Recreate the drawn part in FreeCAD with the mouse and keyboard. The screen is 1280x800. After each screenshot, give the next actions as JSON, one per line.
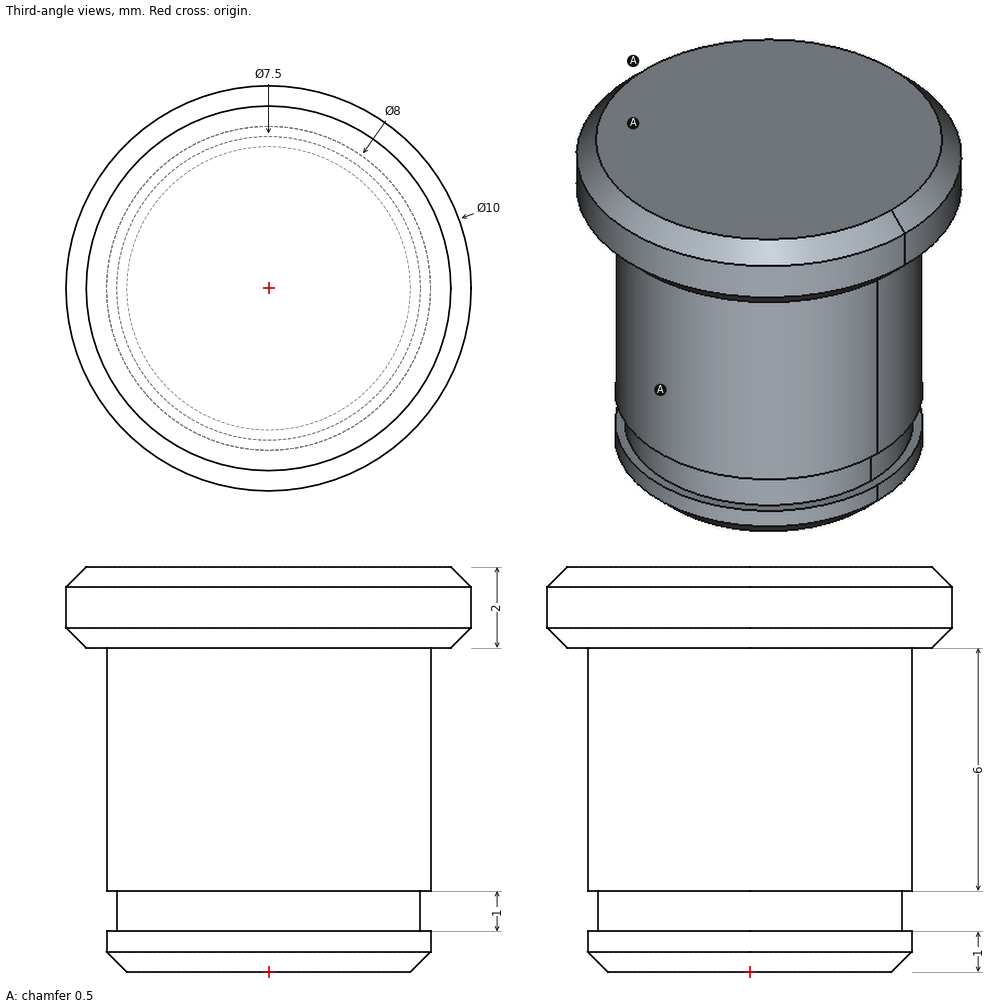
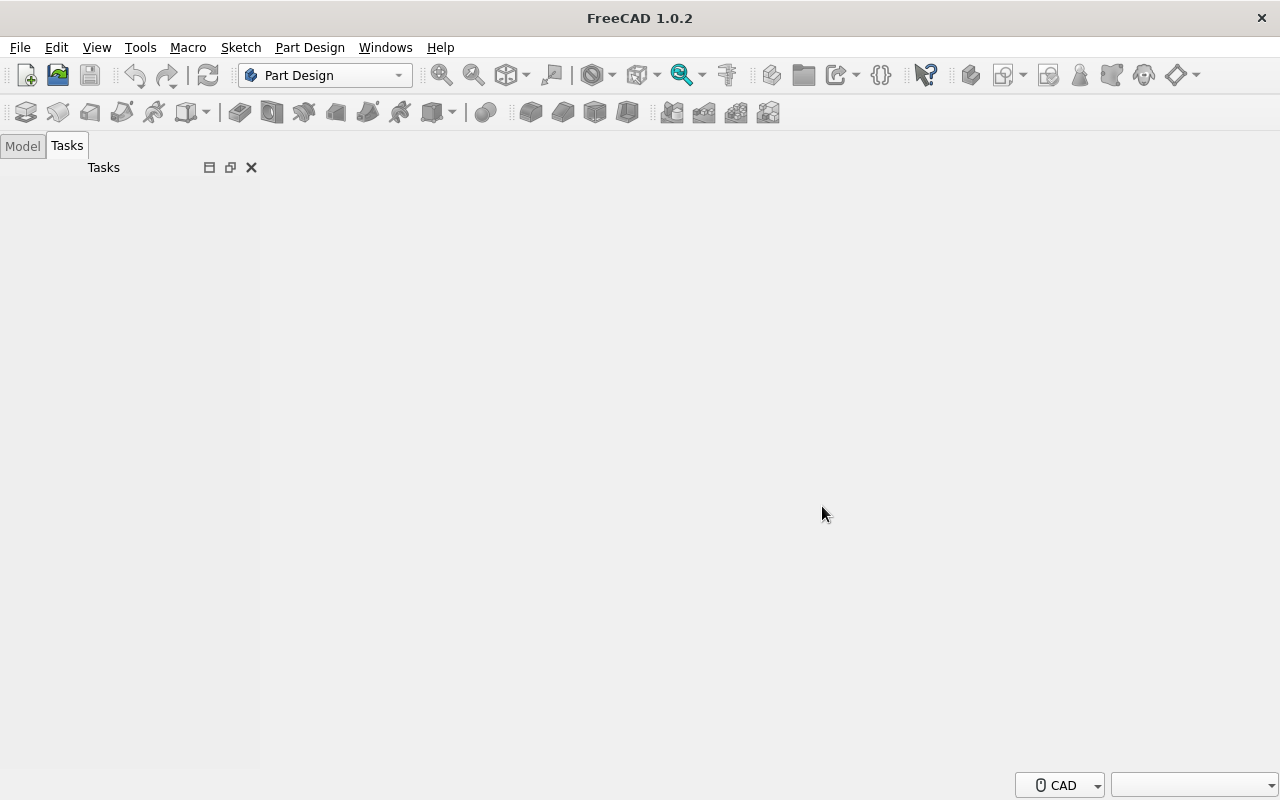
{"action": "key", "text": "ctrl+n"}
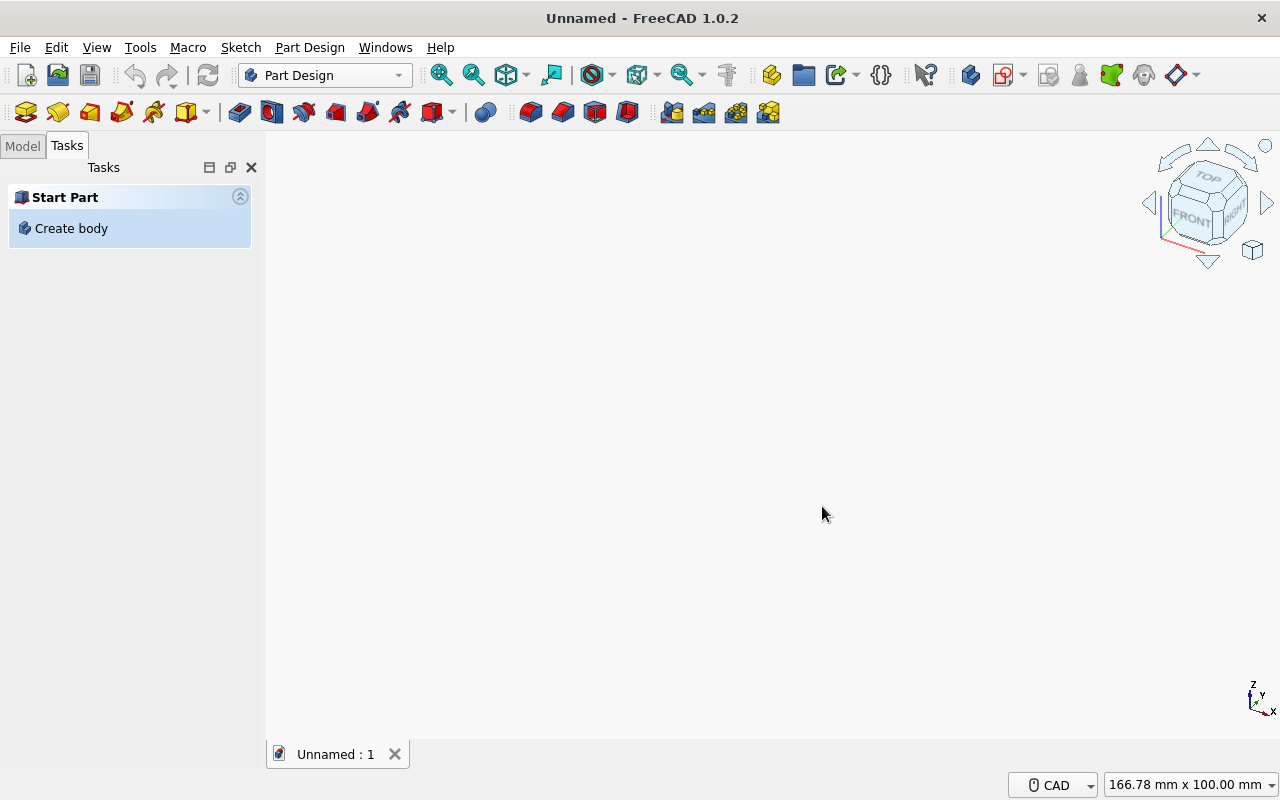
{"action": "left_click", "coordinate": [1004, 76]}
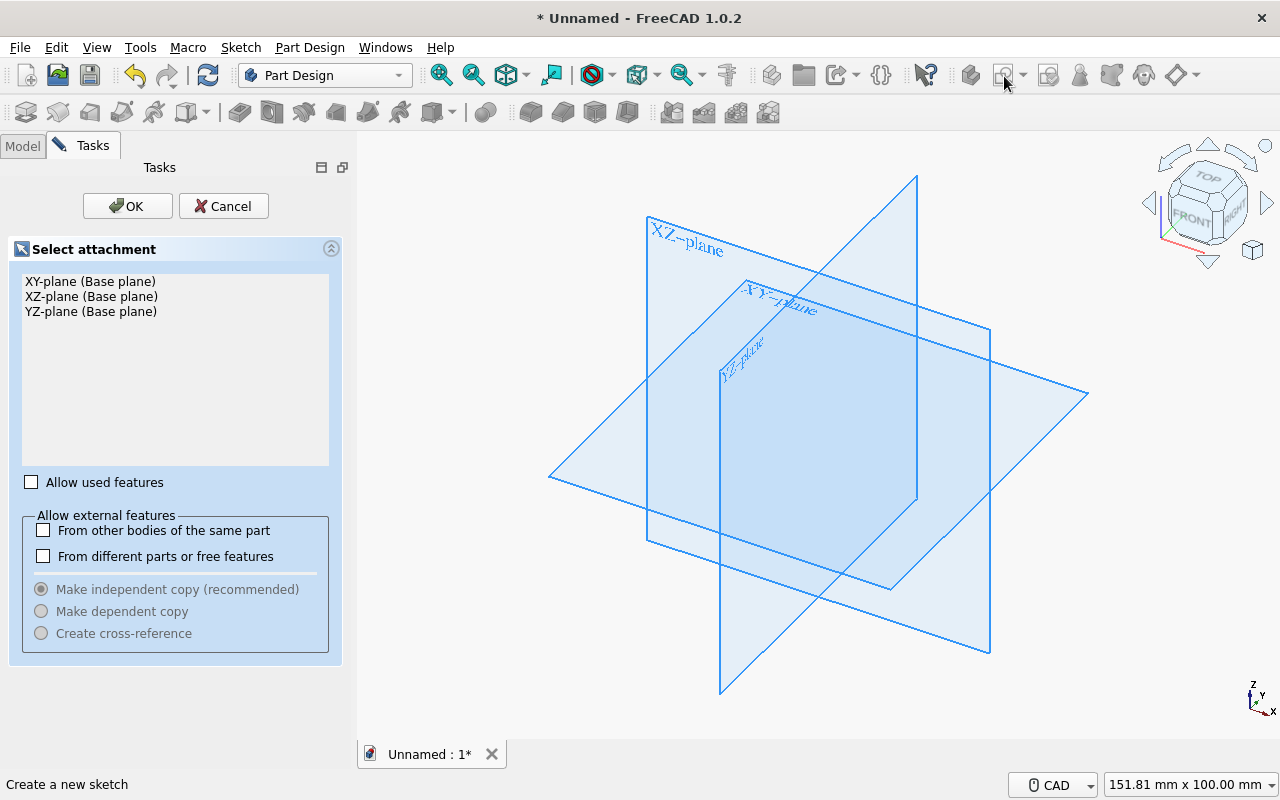
{"action": "left_click", "coordinate": [82, 282]}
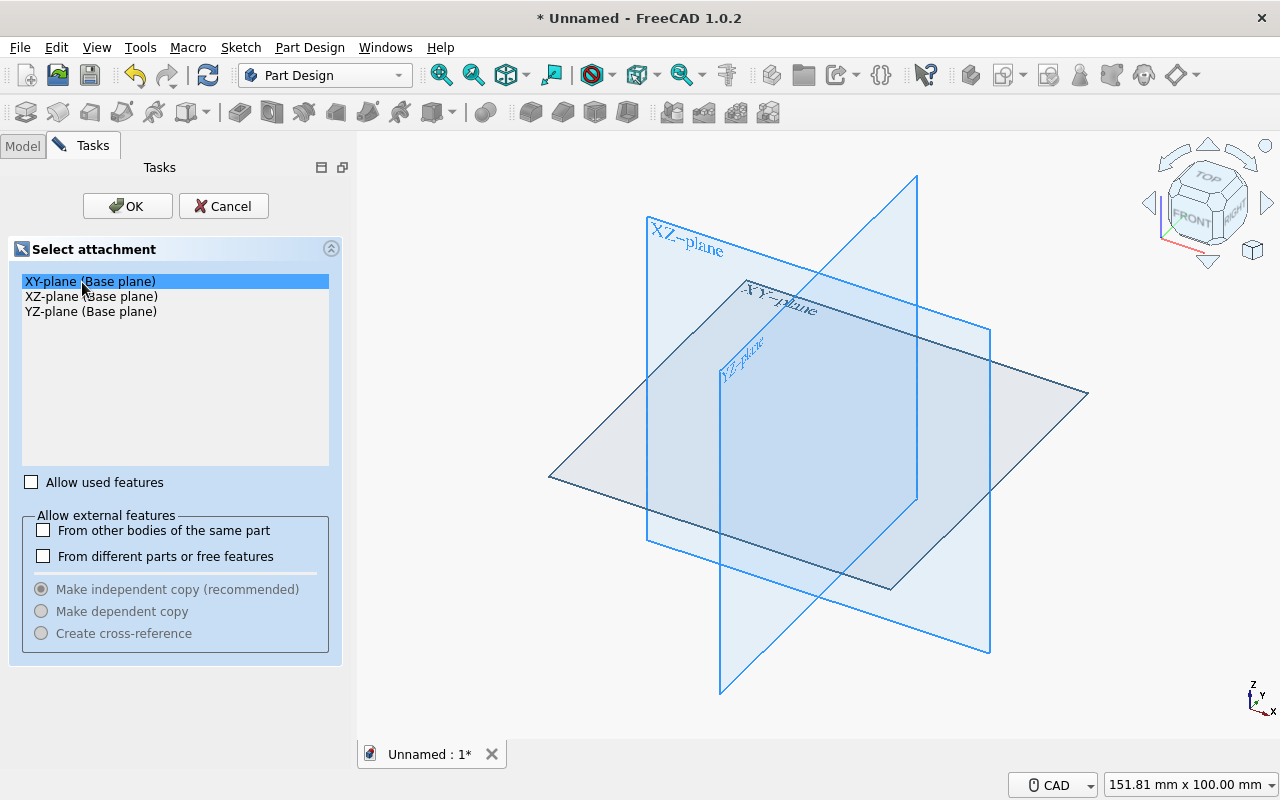
{"action": "left_click", "coordinate": [128, 206]}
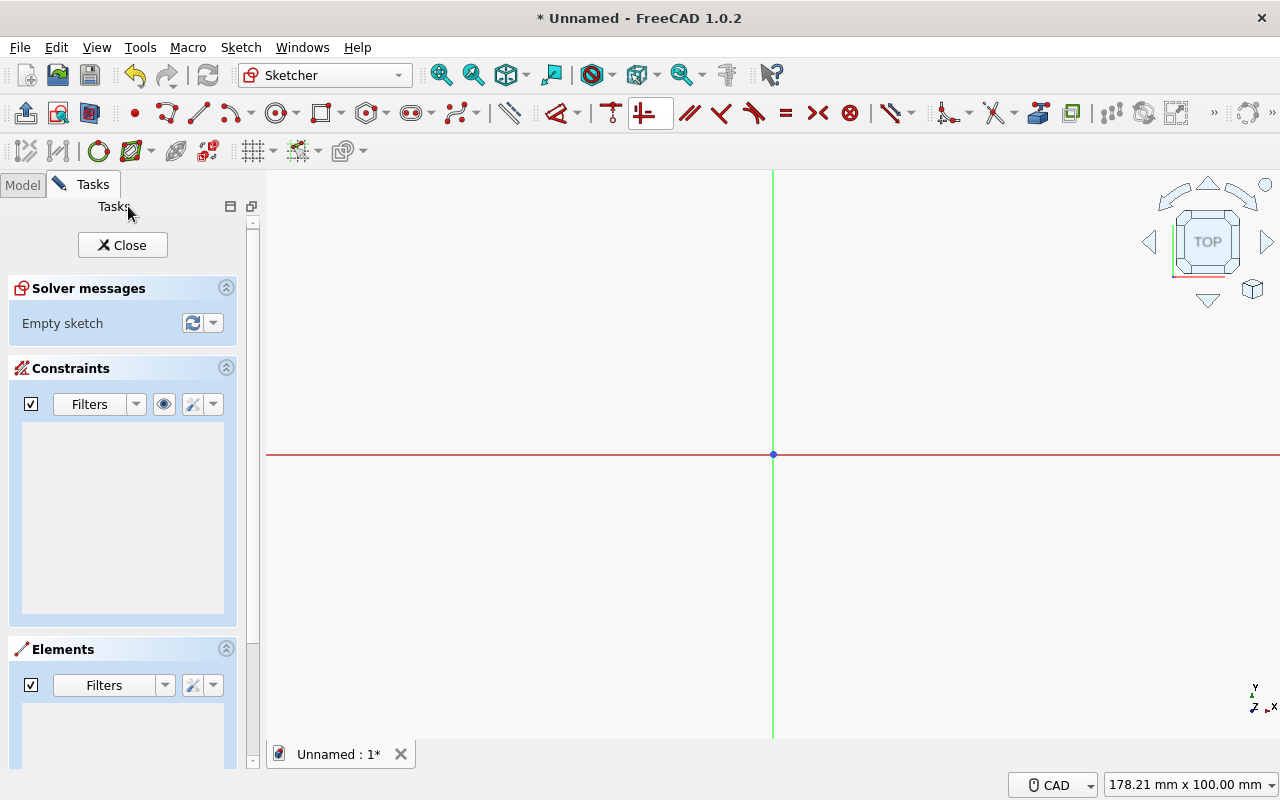
{"action": "scroll", "coordinate": [784, 454], "scroll_direction": "up", "scroll_amount": 10}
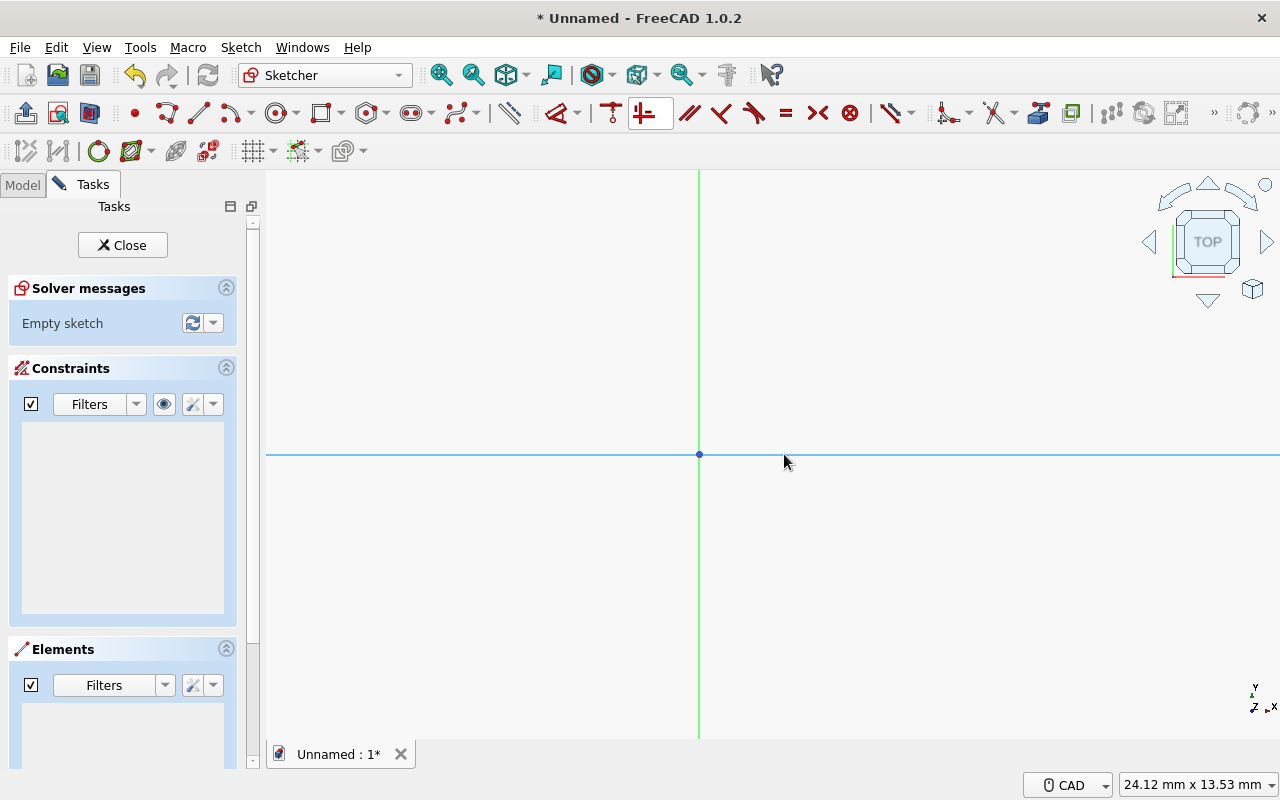
{"action": "left_click", "coordinate": [276, 114]}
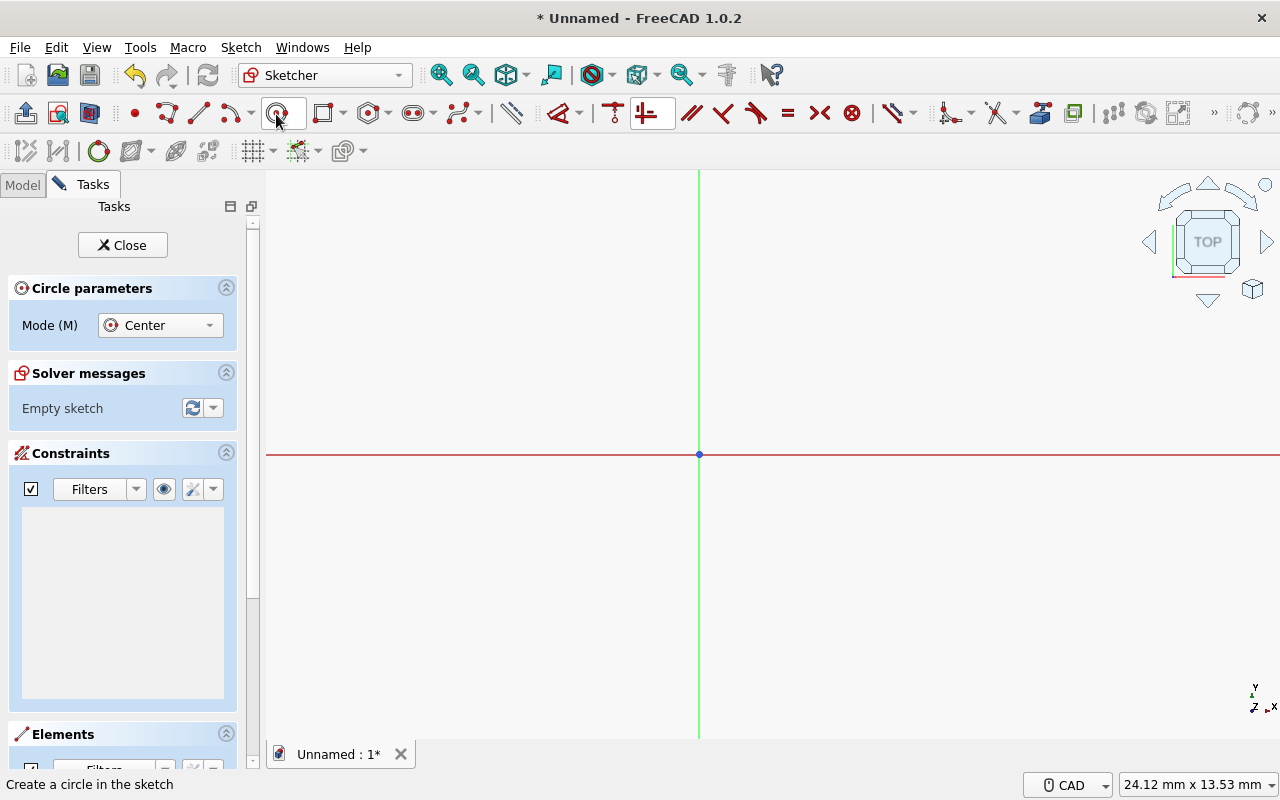
{"action": "left_click", "coordinate": [699, 454]}
{"action": "left_click", "coordinate": [818, 336]}
{"action": "key", "text": "Escape"}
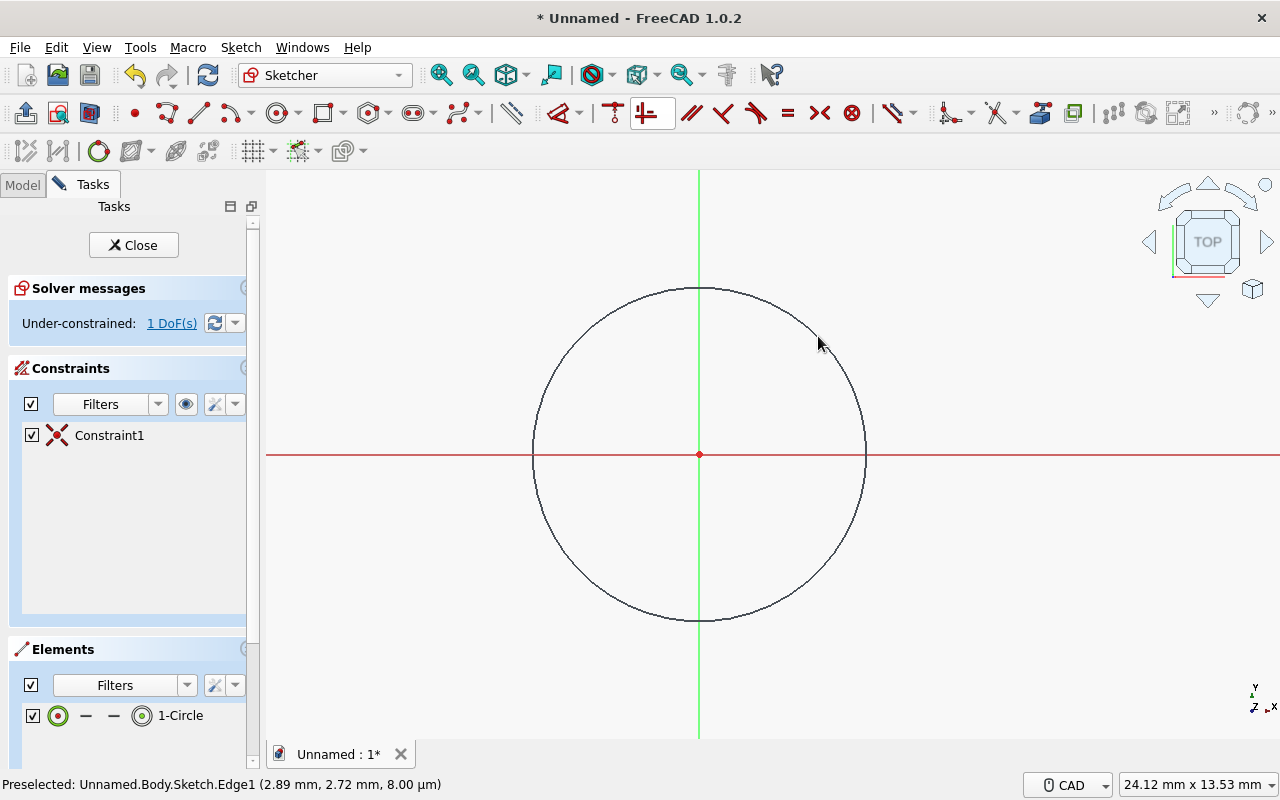
{"action": "key", "text": "d"}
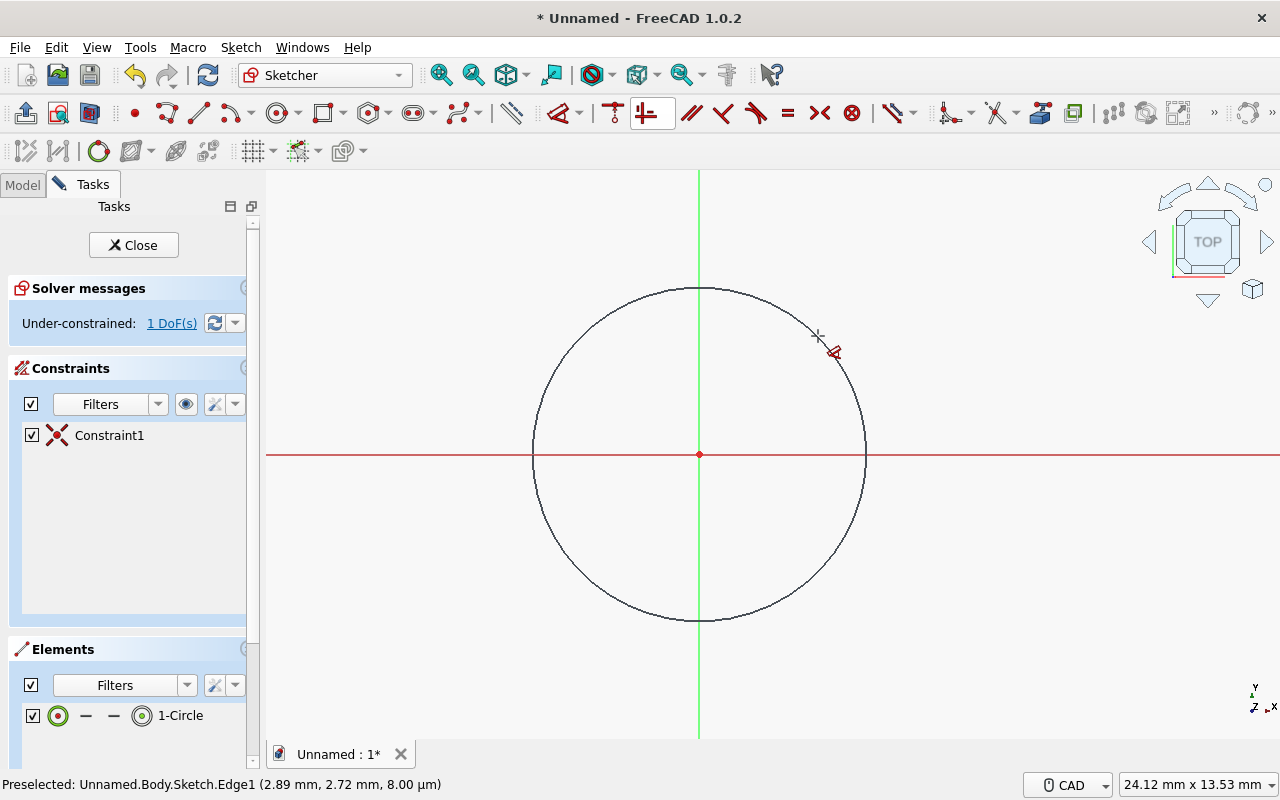
{"action": "left_click", "coordinate": [817, 336]}
{"action": "left_click", "coordinate": [840, 313]}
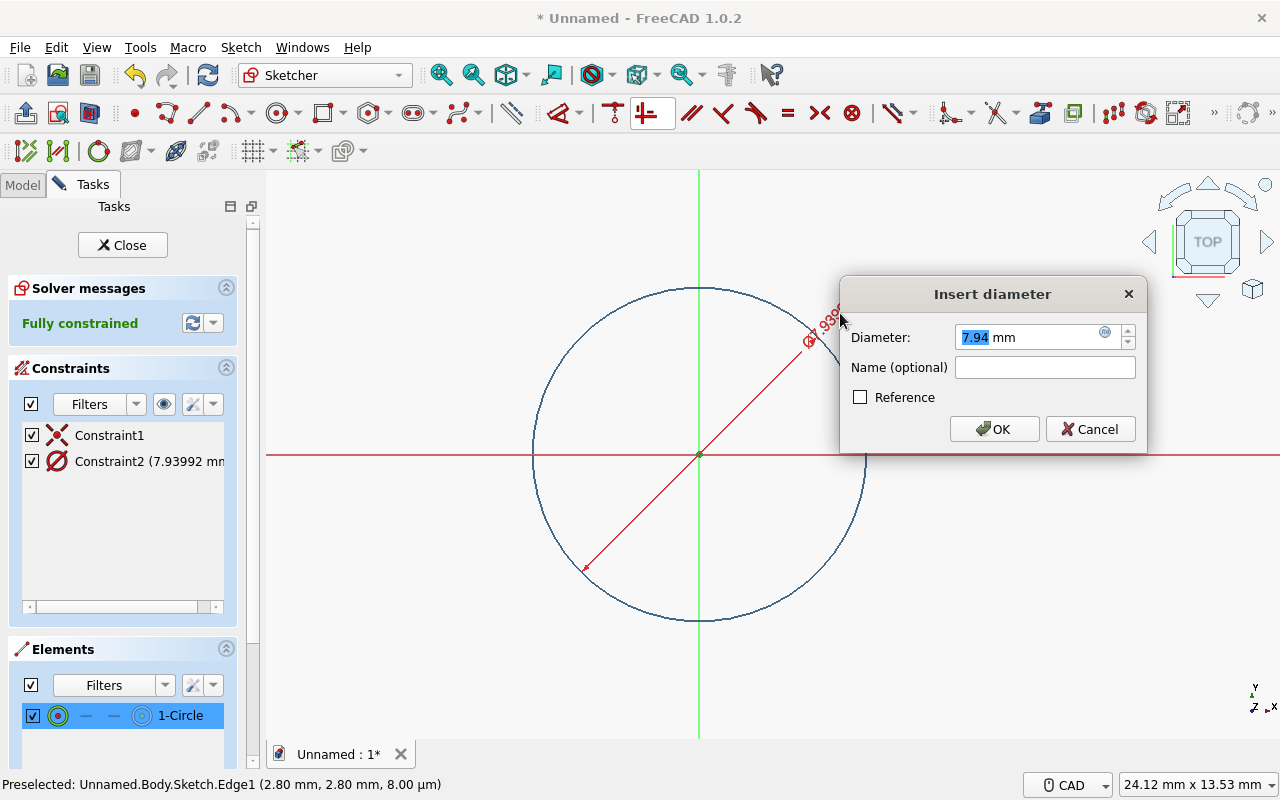
{"action": "type", "text": "8"}
{"action": "key", "text": "Return"}
{"action": "key", "text": "Escape"}